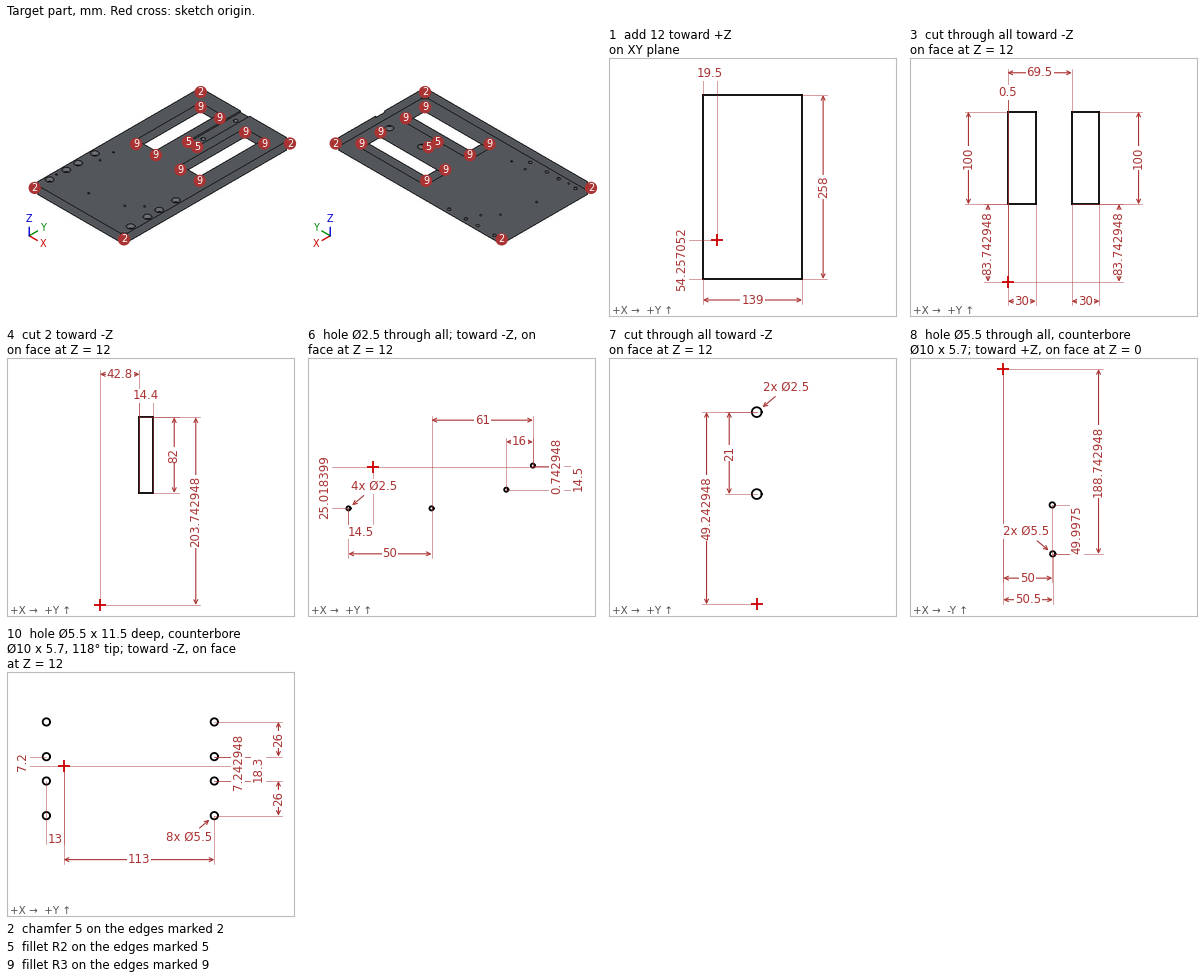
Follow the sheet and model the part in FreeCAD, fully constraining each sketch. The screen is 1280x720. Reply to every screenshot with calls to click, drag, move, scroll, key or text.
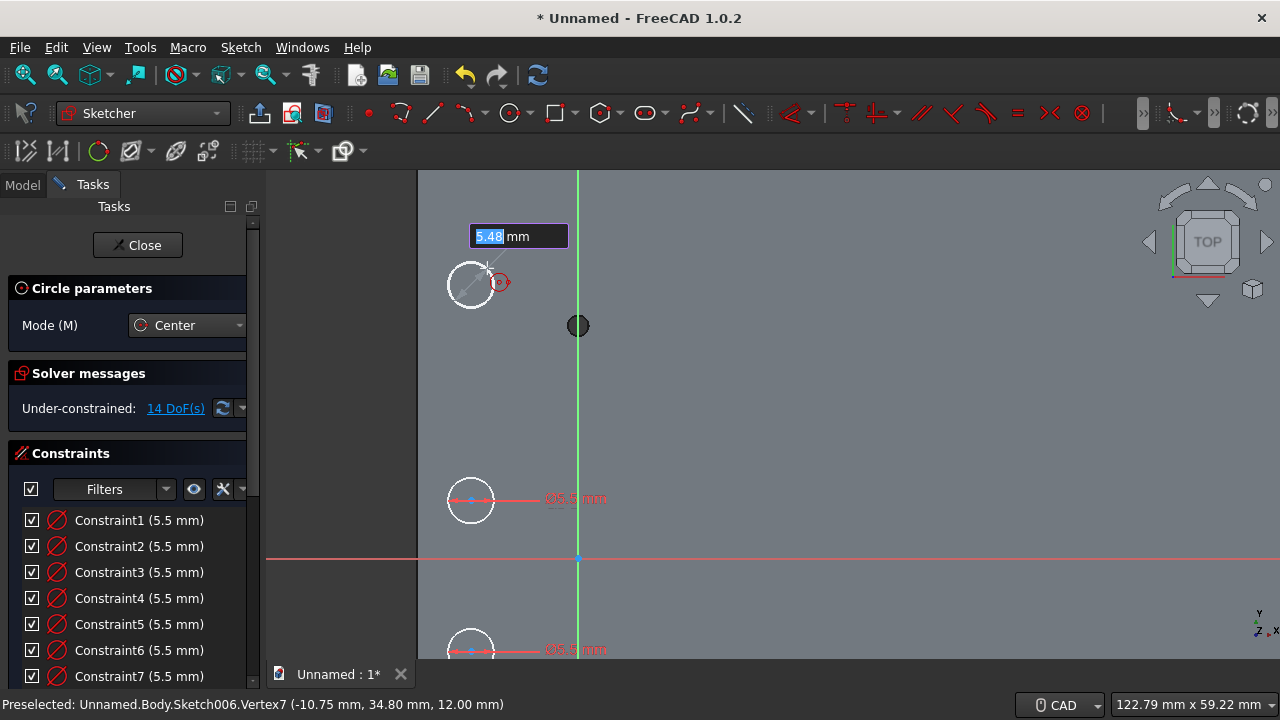
text(5.5)
key(Return)
key(Escape)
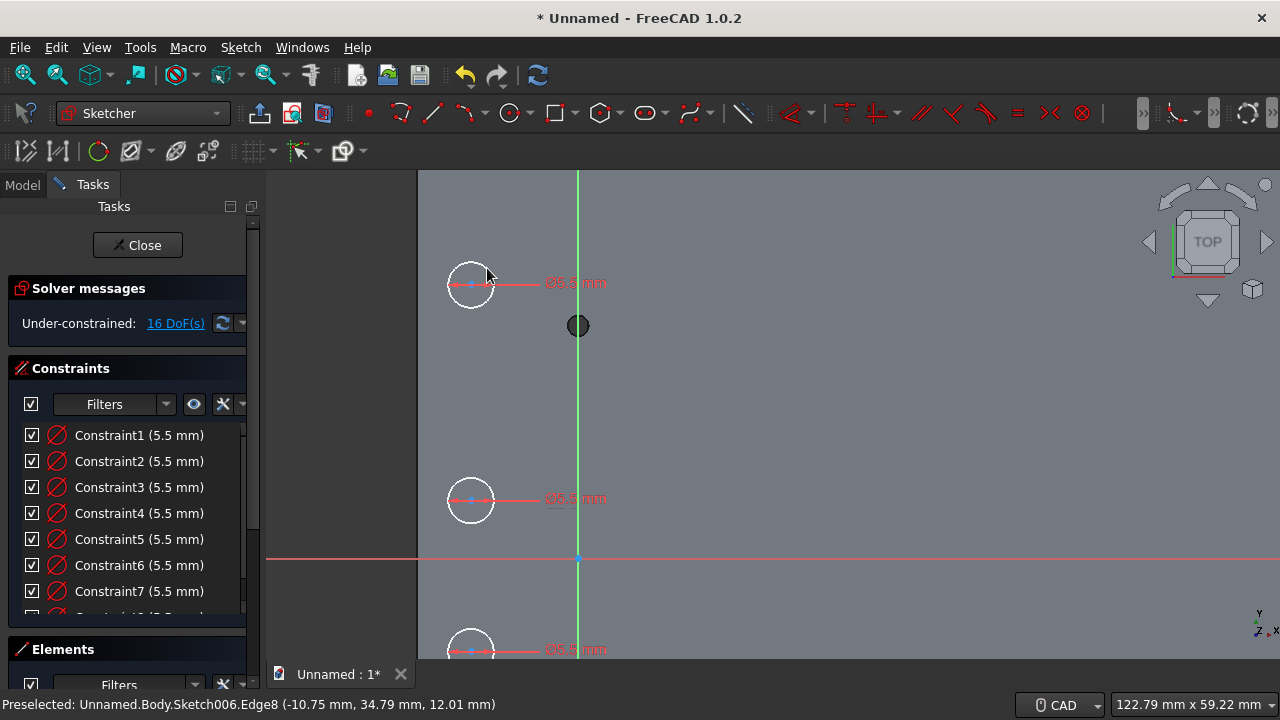
scroll(471, 284, down, 4)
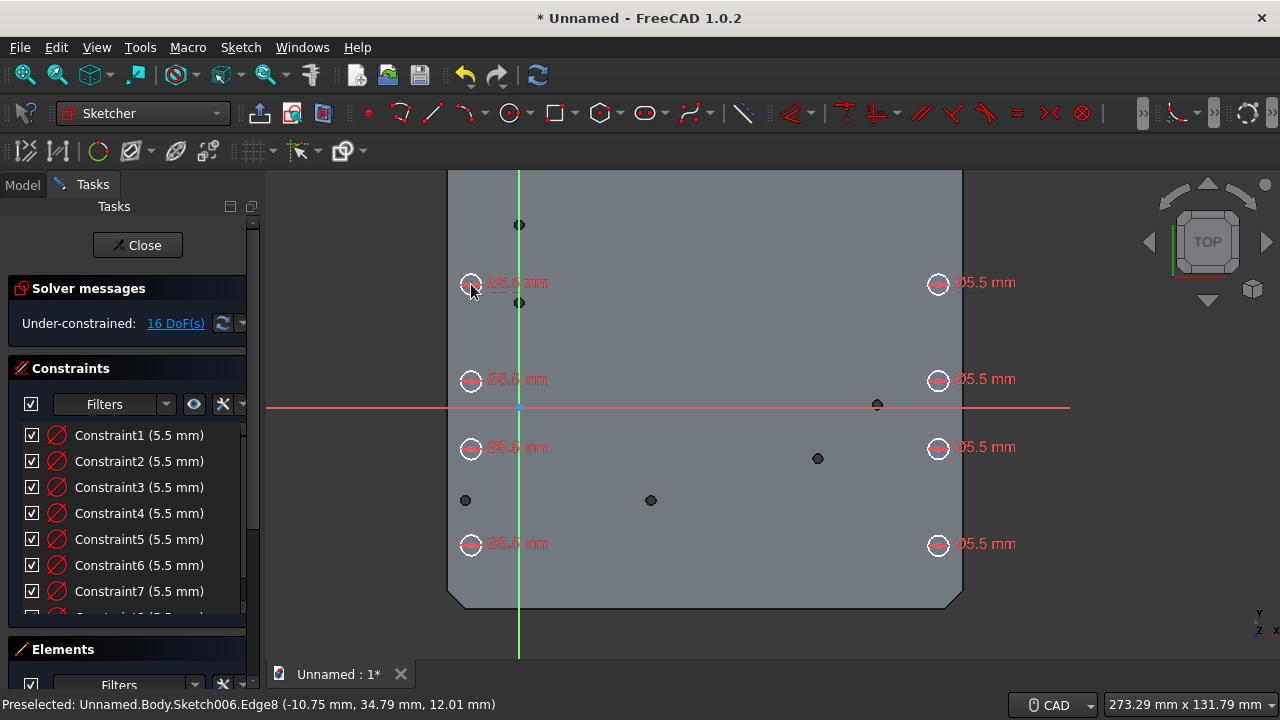
click(938, 546)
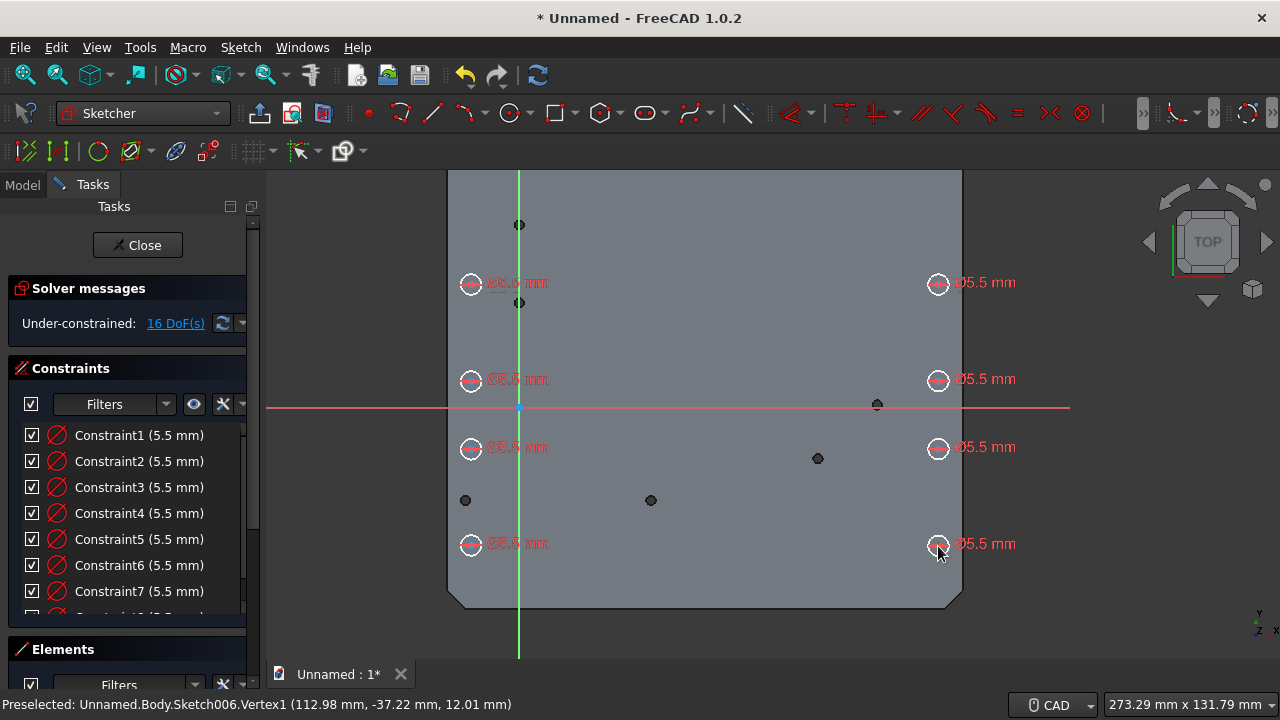
click(938, 449)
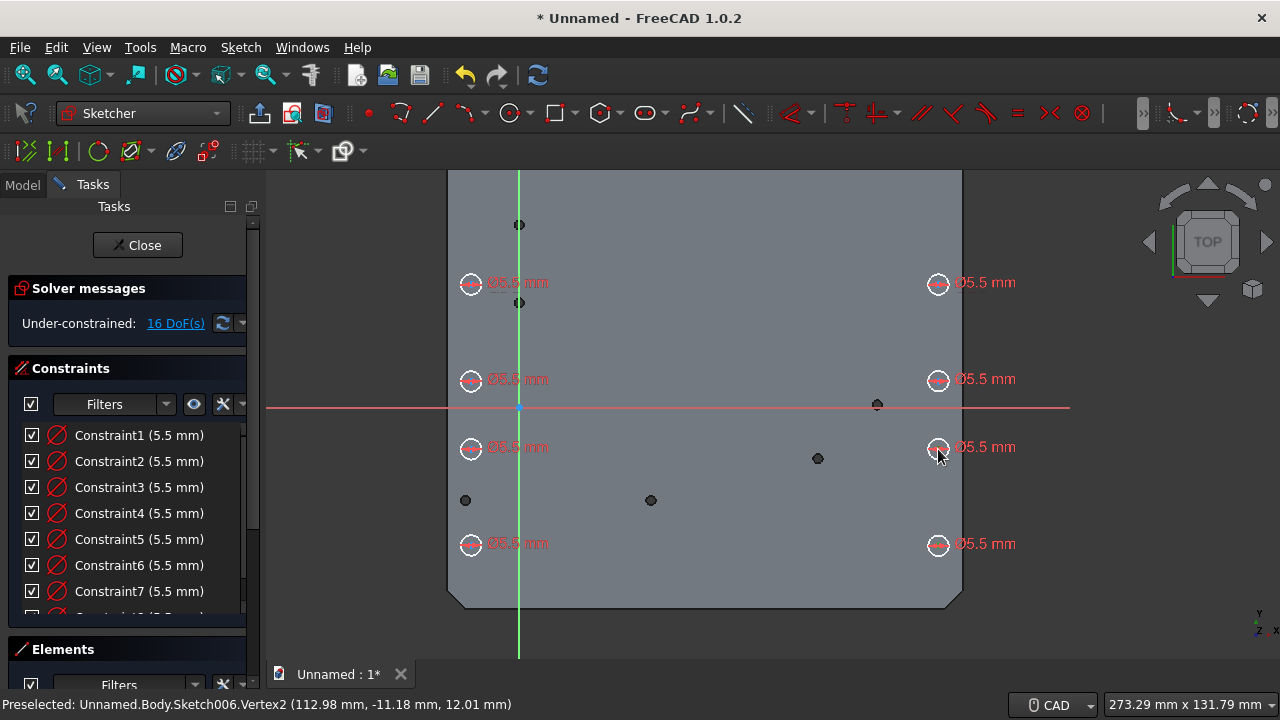
click(900, 114)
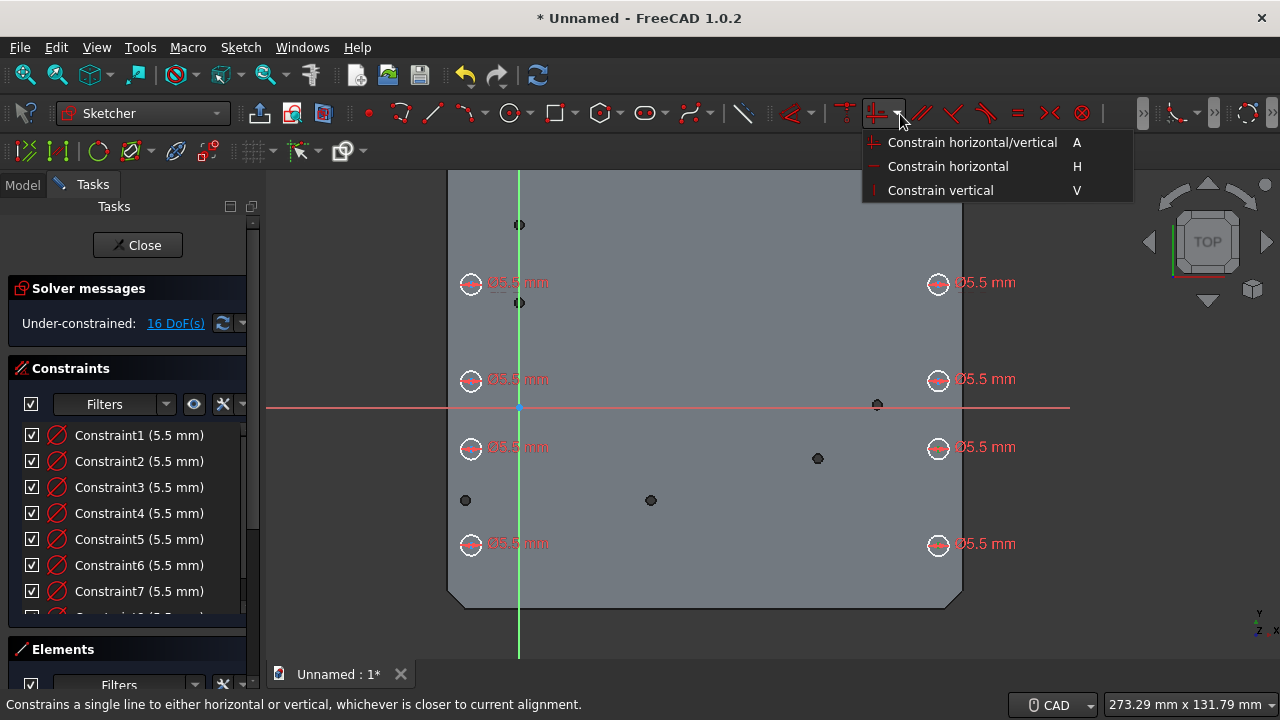
click(998, 190)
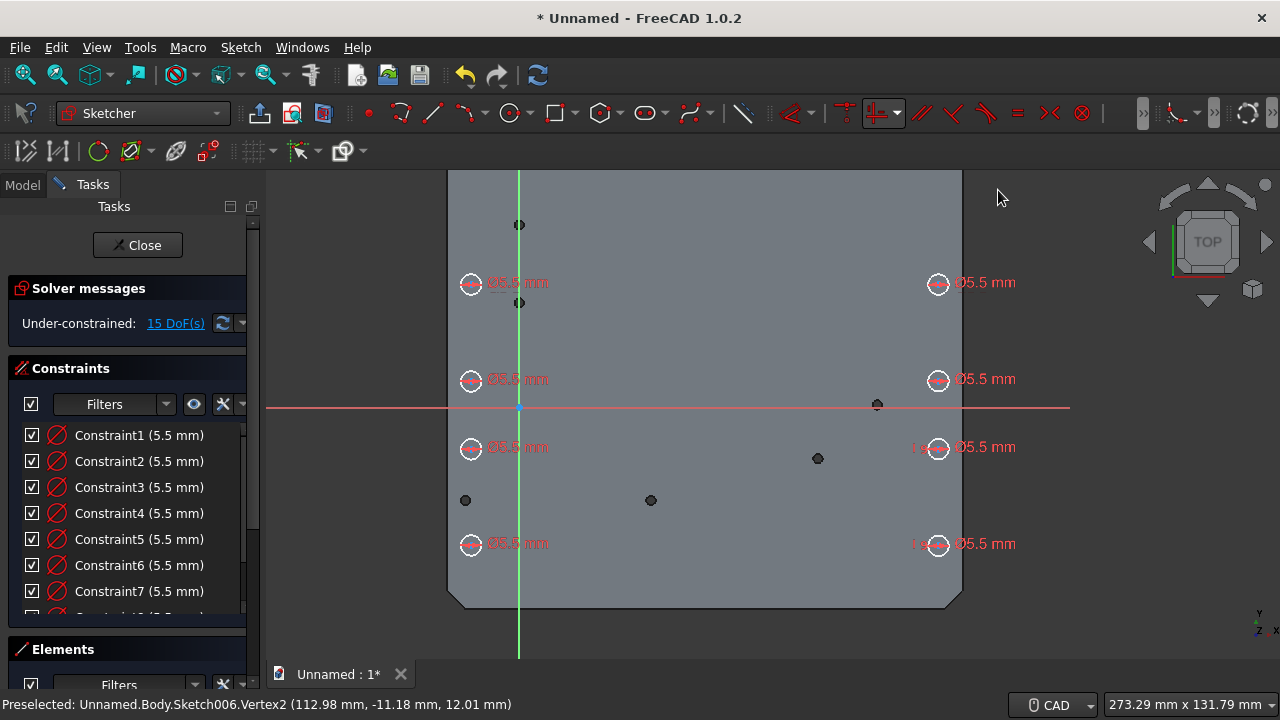
click(938, 449)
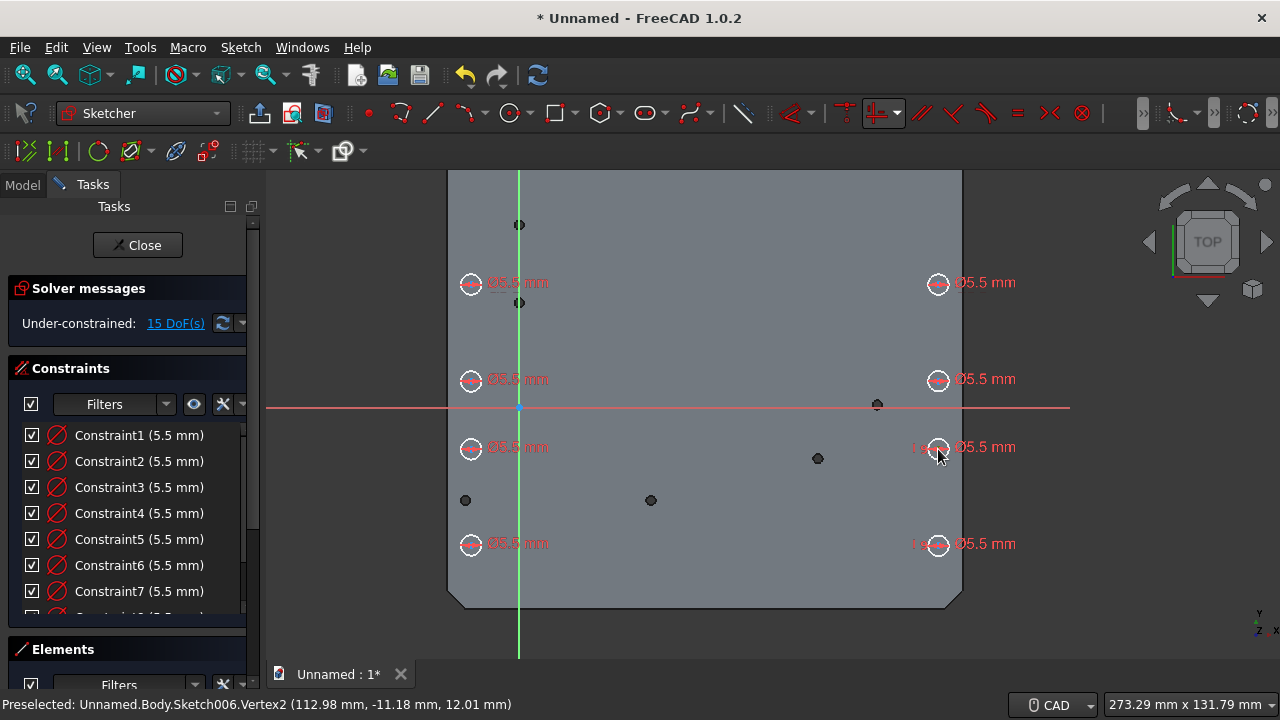
click(938, 381)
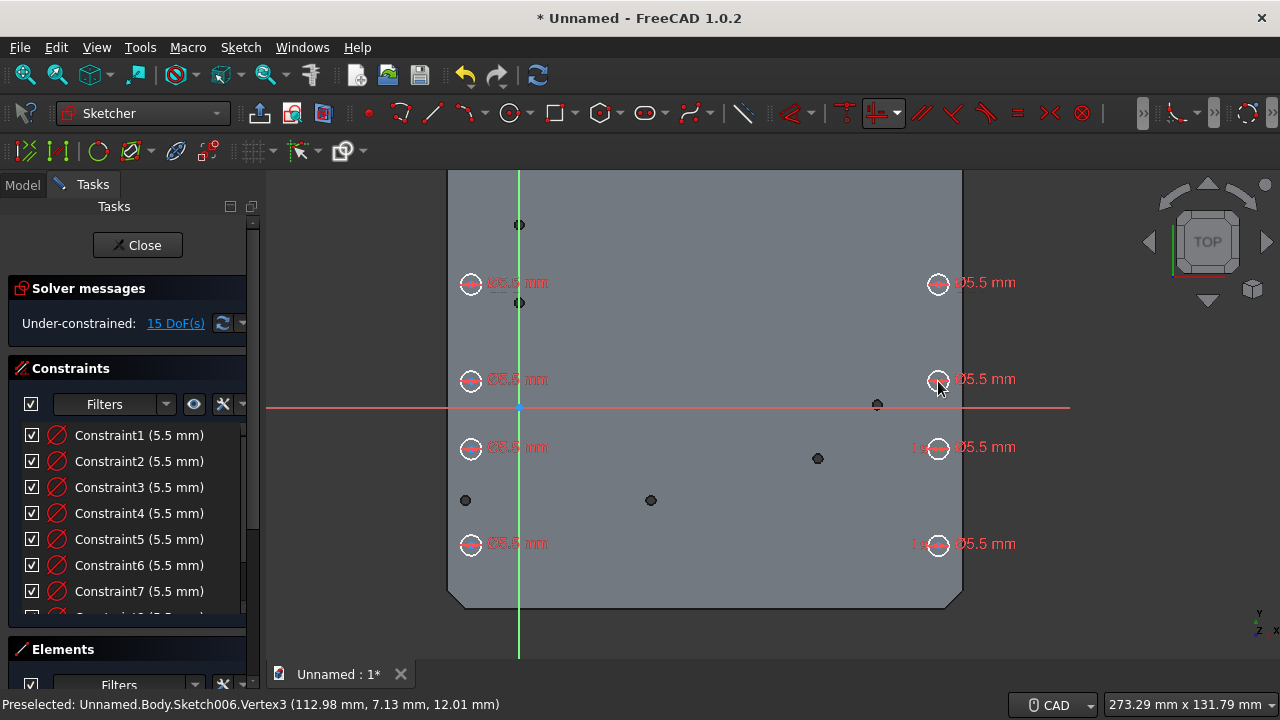
key(v)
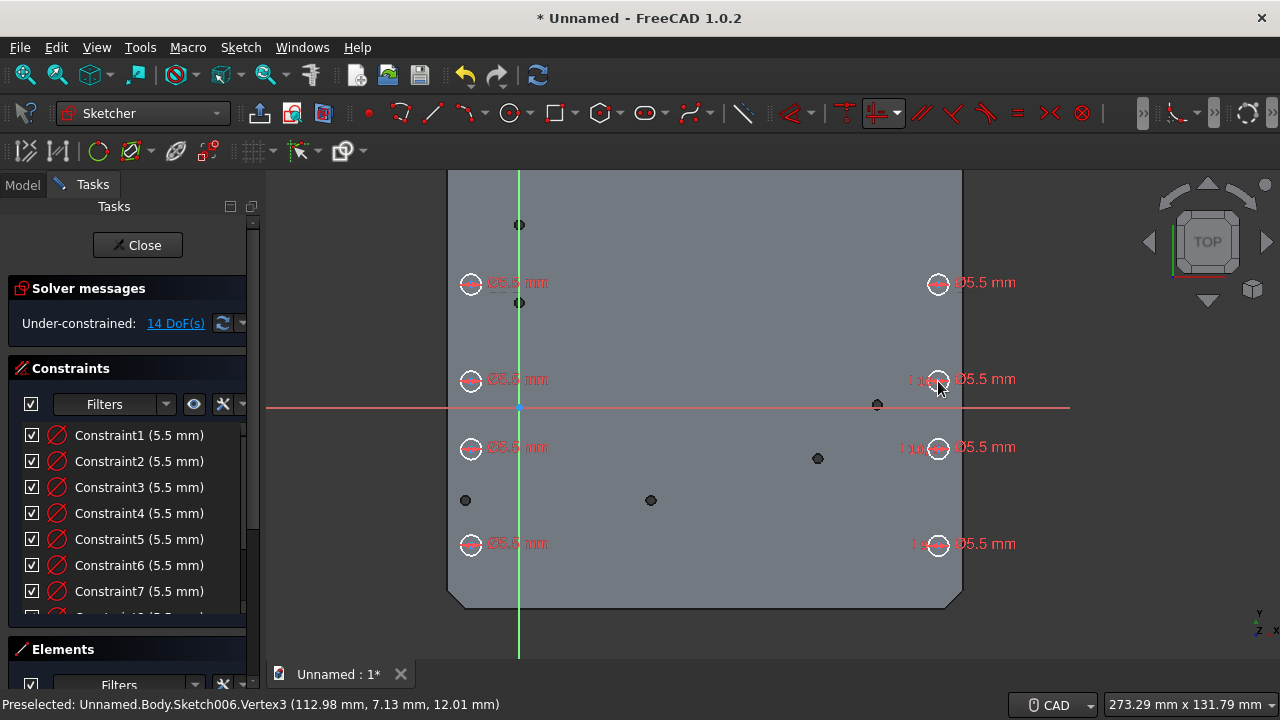
click(938, 381)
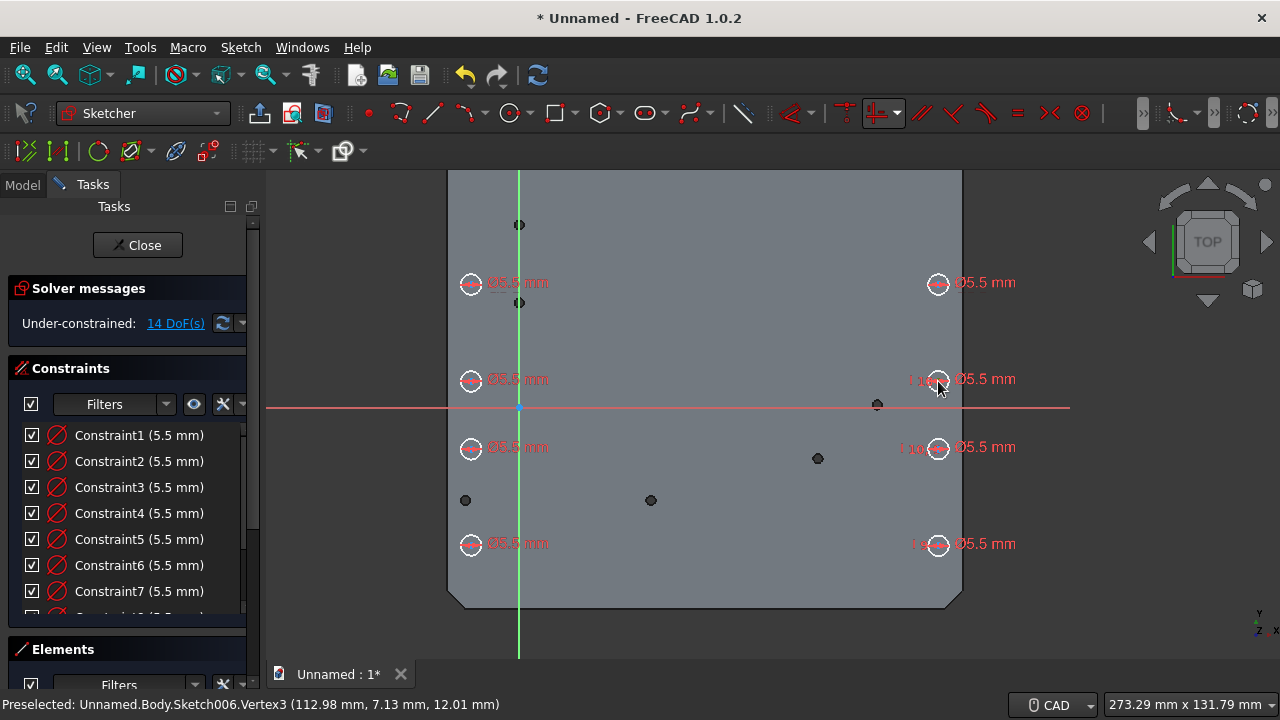
click(938, 285)